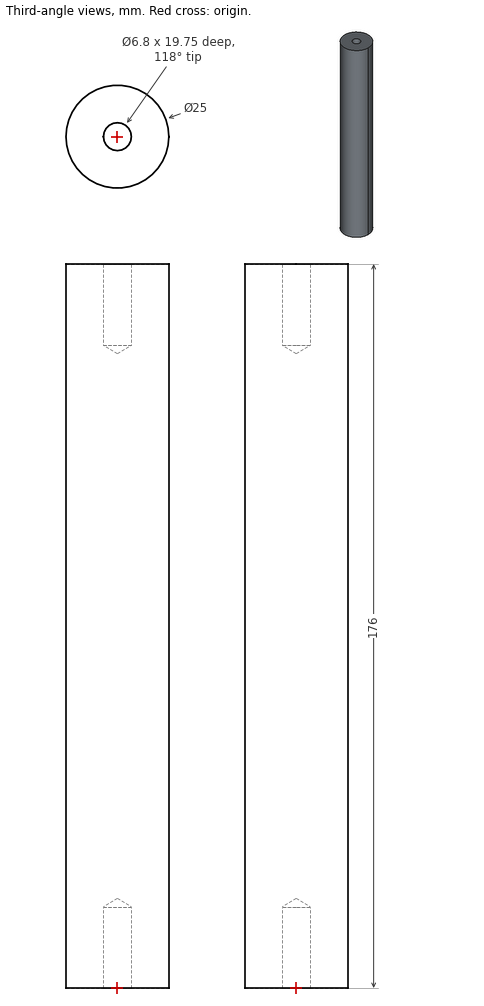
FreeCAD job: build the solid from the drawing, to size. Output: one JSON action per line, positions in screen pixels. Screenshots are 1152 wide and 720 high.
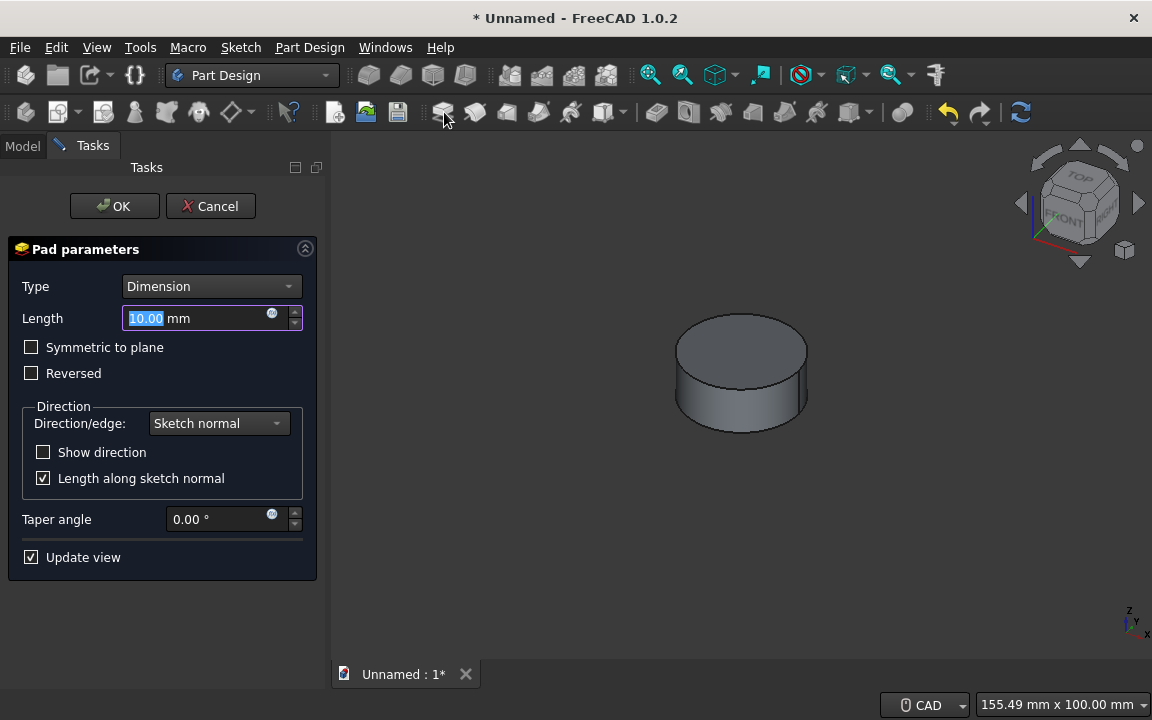
{"action": "type", "text": "176"}
{"action": "key", "text": "Tab"}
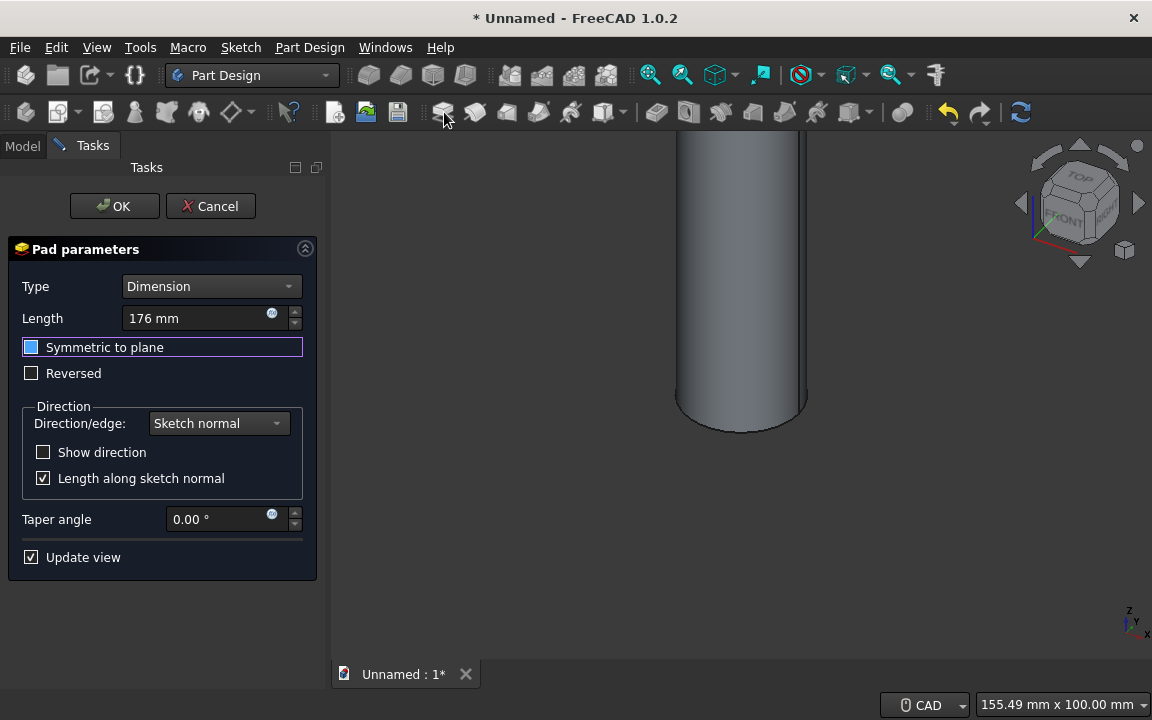
{"action": "left_click", "coordinate": [115, 206]}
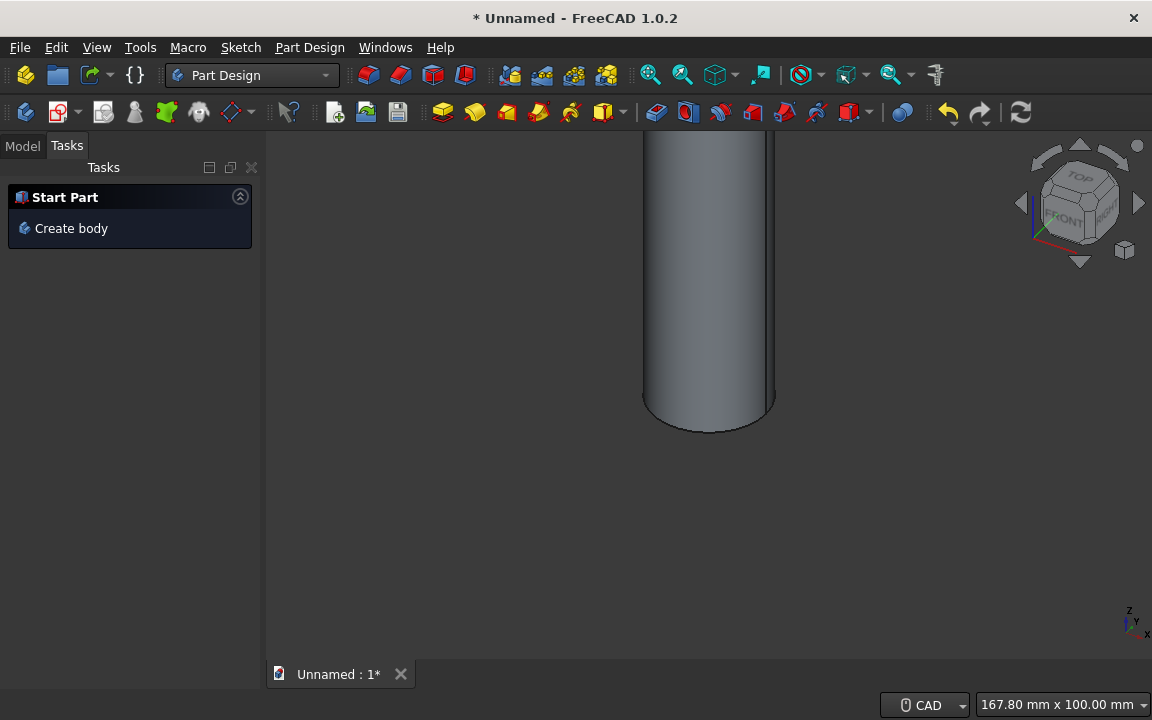
{"action": "key", "text": "v f"}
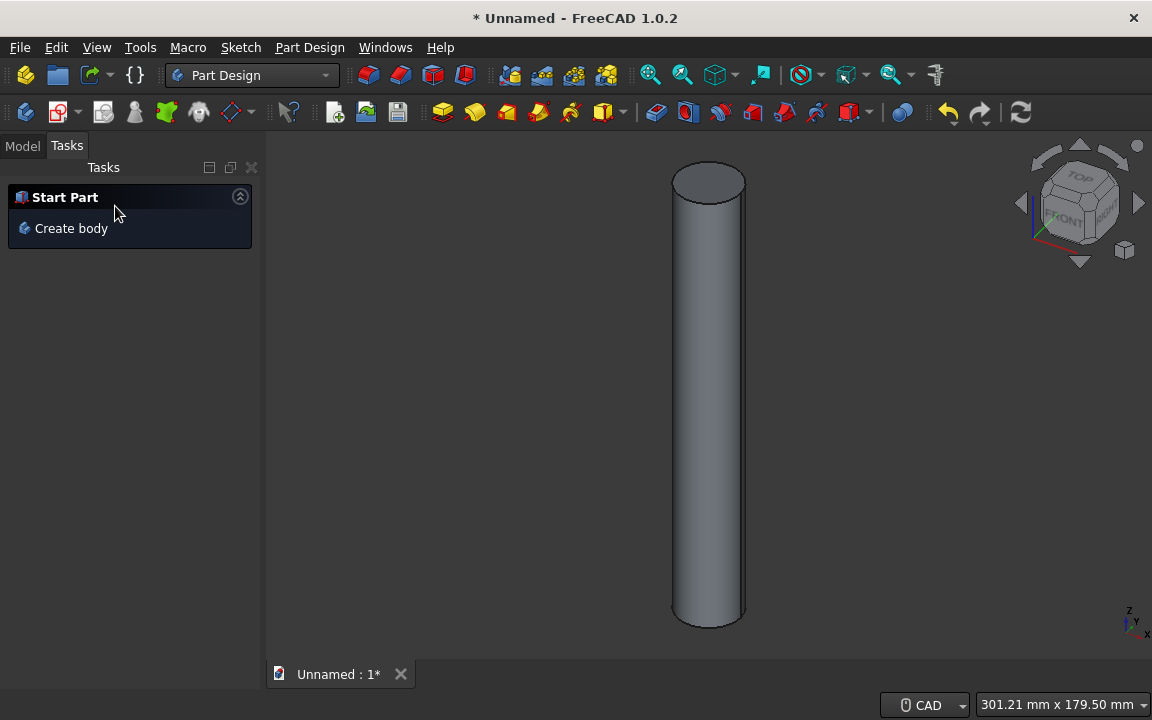
{"action": "left_click", "coordinate": [58, 112]}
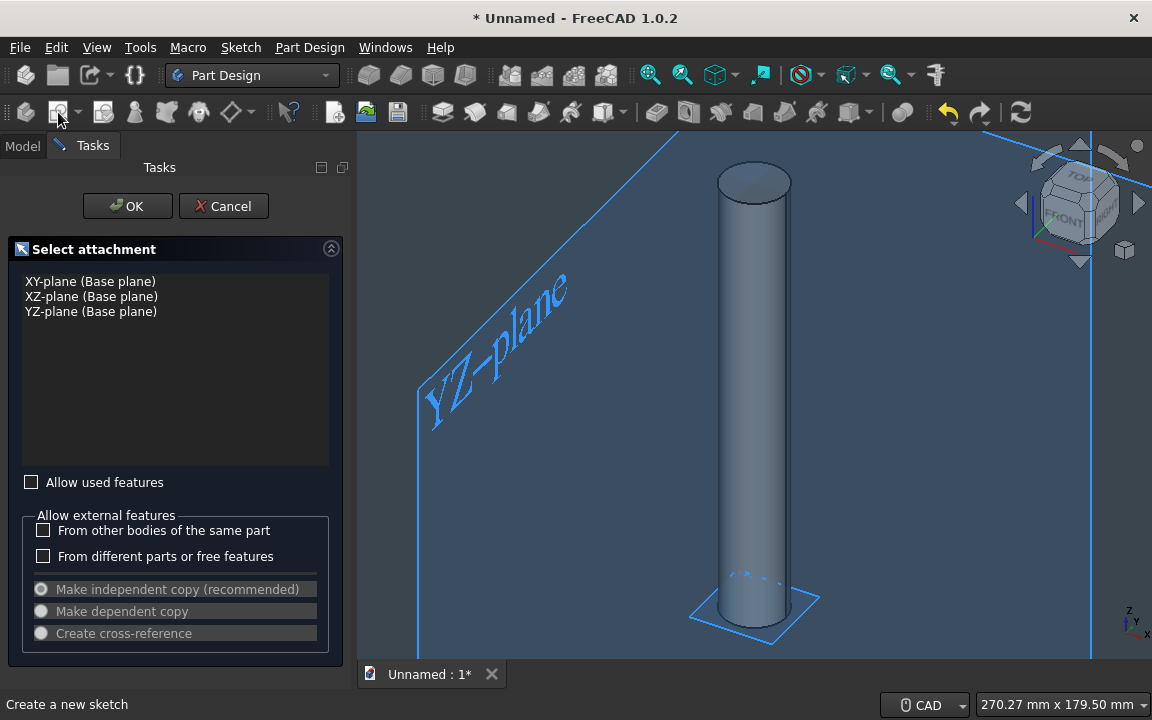
{"action": "left_click", "coordinate": [82, 282]}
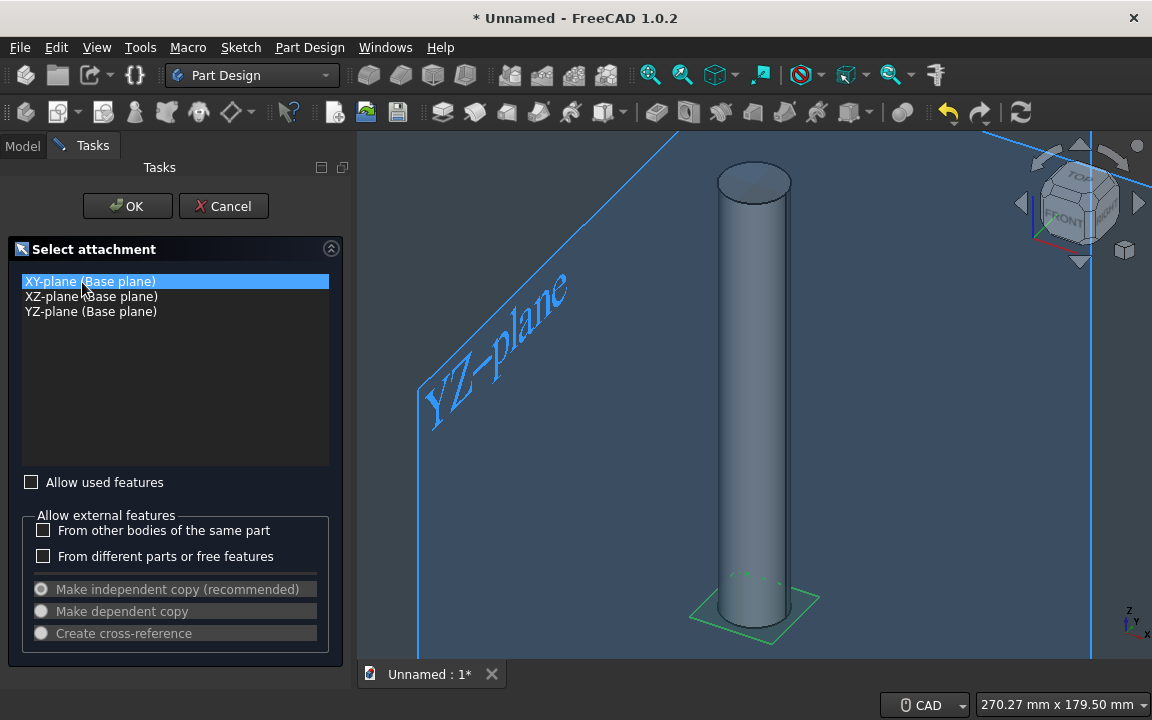
{"action": "left_click", "coordinate": [128, 206]}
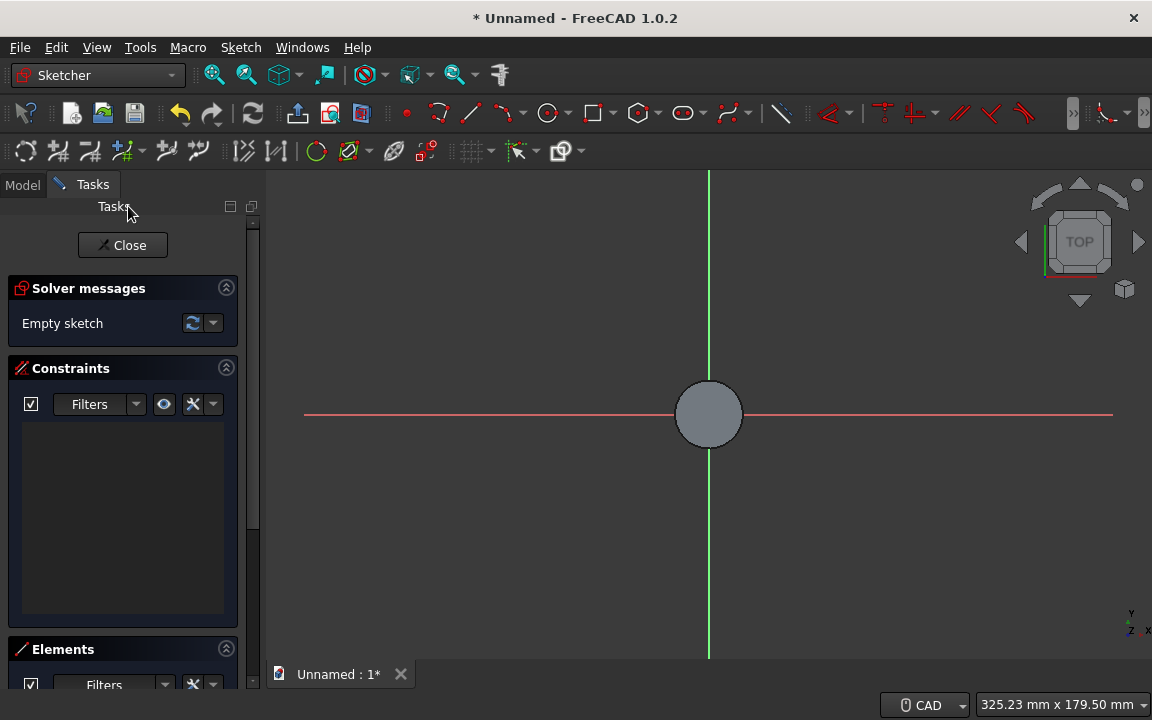
{"action": "key", "text": "q s"}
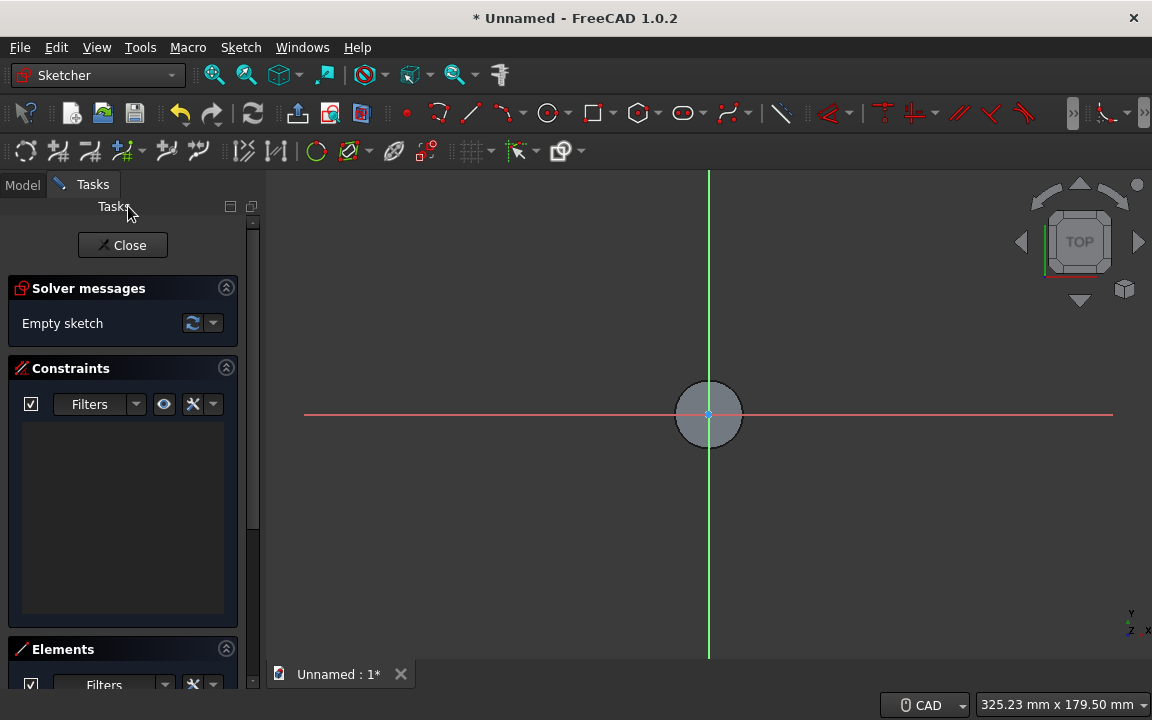
{"action": "scroll", "coordinate": [713, 414], "scroll_direction": "up", "scroll_amount": 14}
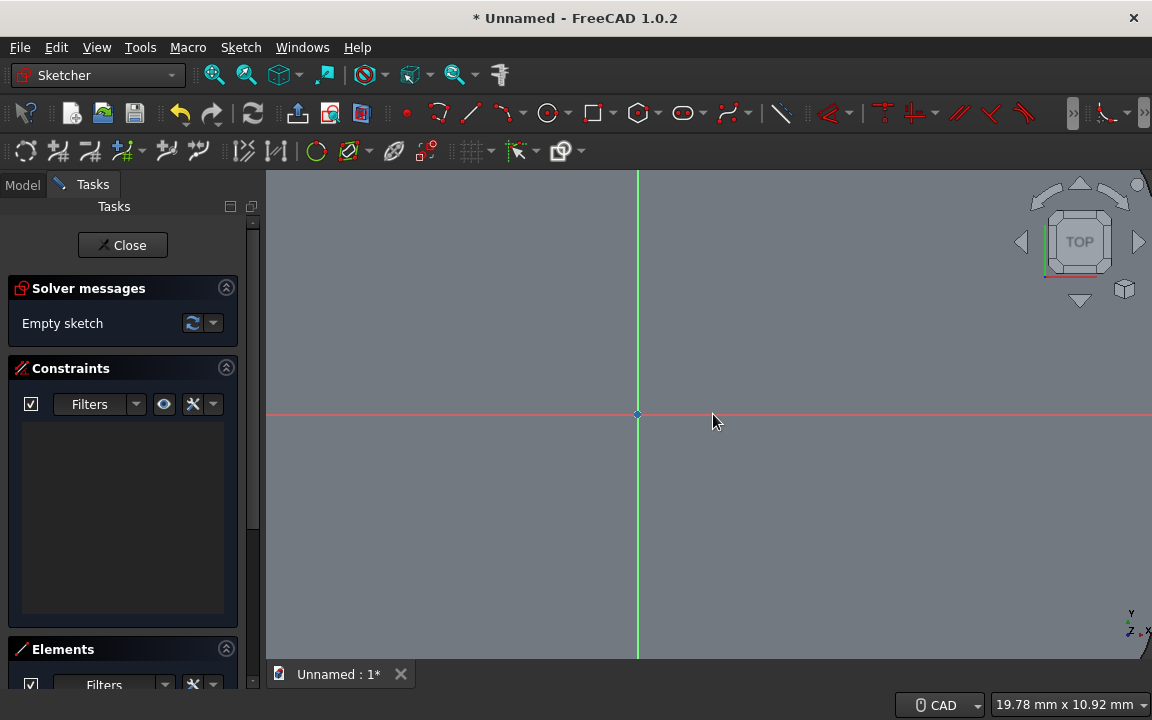
{"action": "key", "text": "g c"}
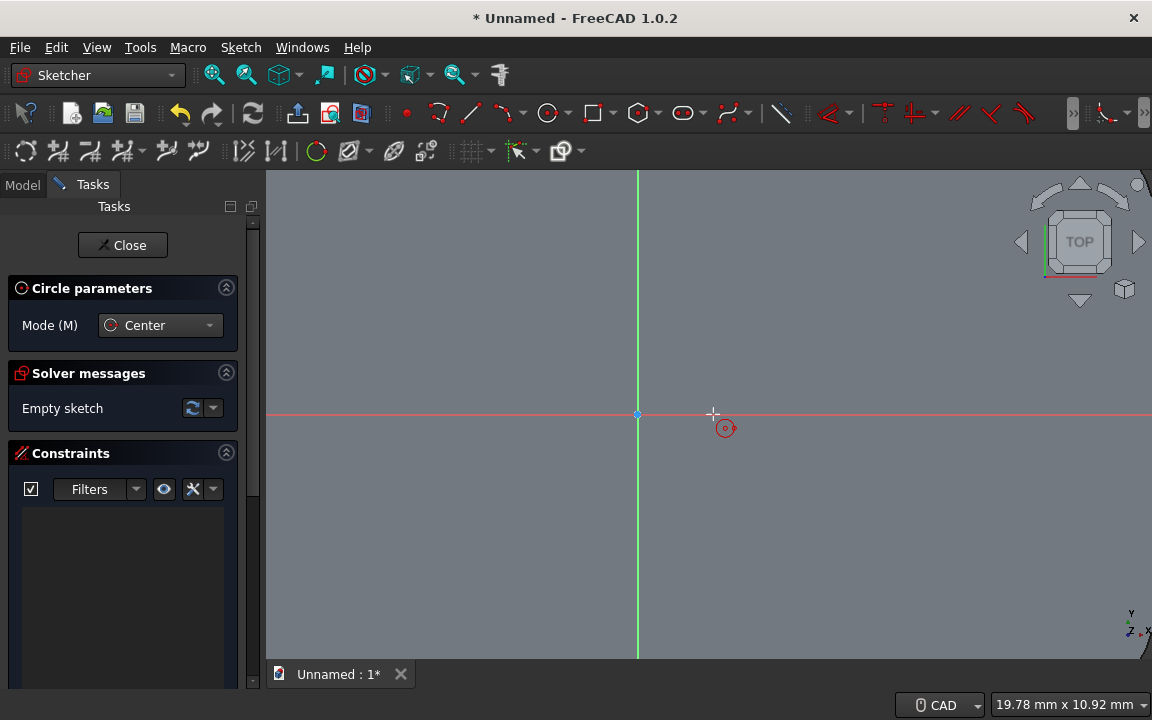
{"action": "left_click", "coordinate": [638, 414]}
{"action": "left_click", "coordinate": [745, 307]}
{"action": "key", "text": "Escape"}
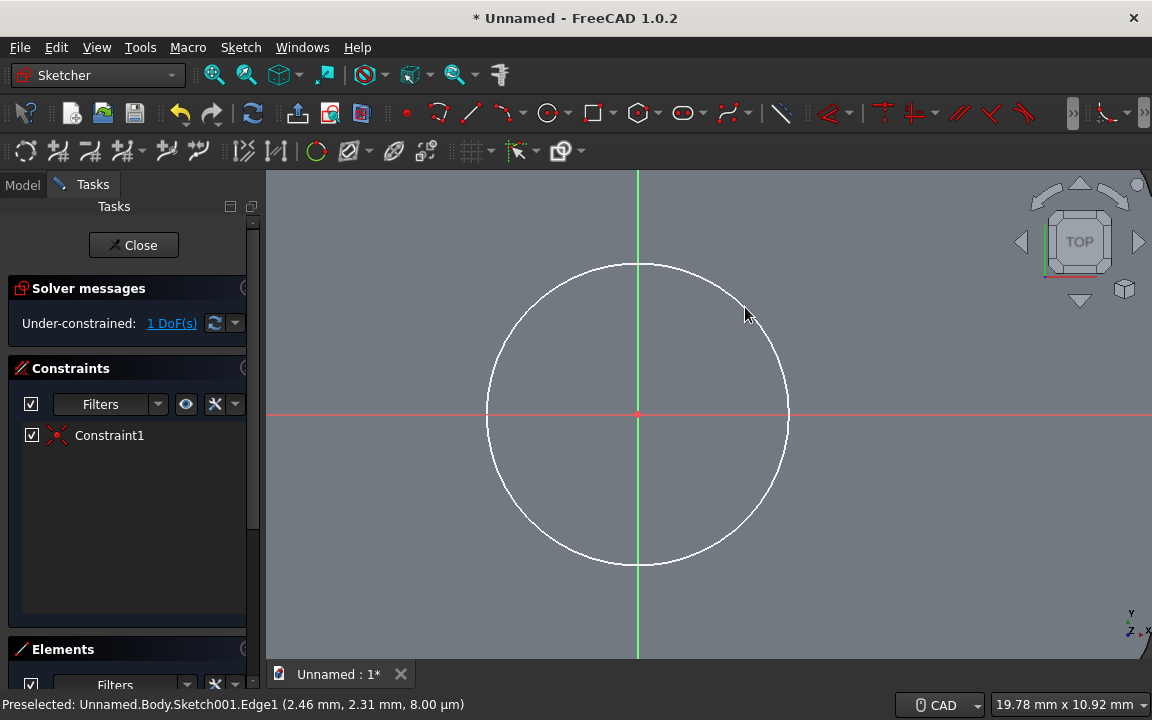
{"action": "left_click", "coordinate": [828, 114]}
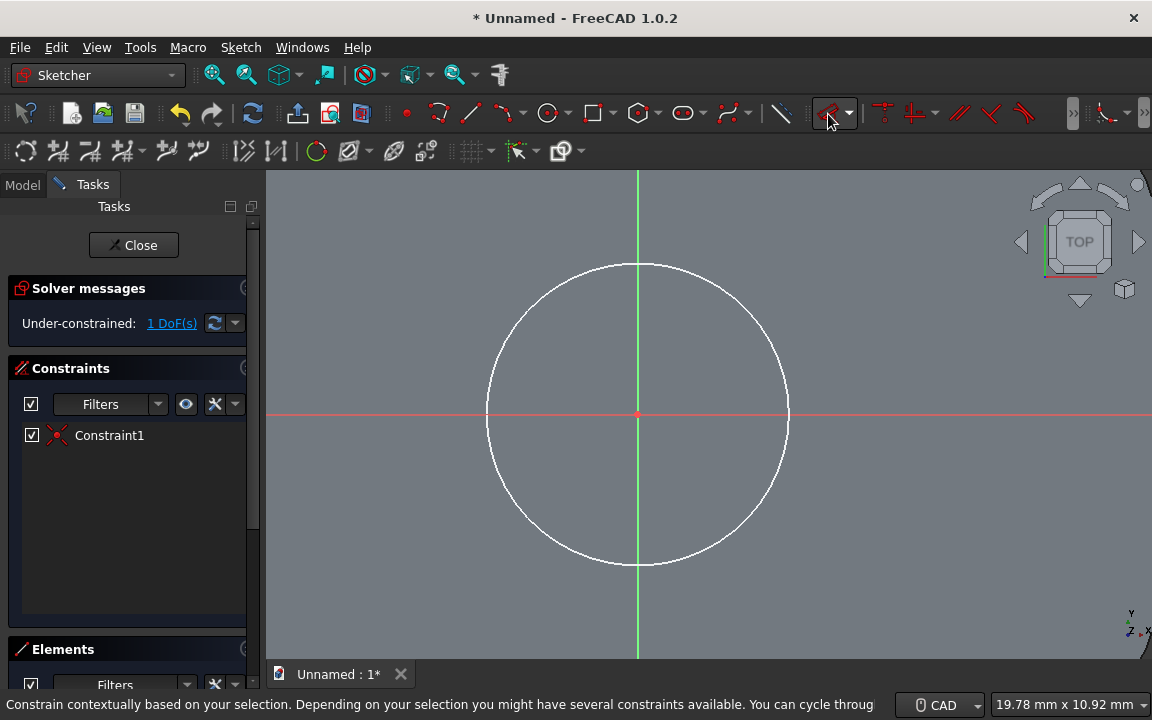
{"action": "left_click", "coordinate": [744, 307]}
{"action": "left_click", "coordinate": [766, 284]}